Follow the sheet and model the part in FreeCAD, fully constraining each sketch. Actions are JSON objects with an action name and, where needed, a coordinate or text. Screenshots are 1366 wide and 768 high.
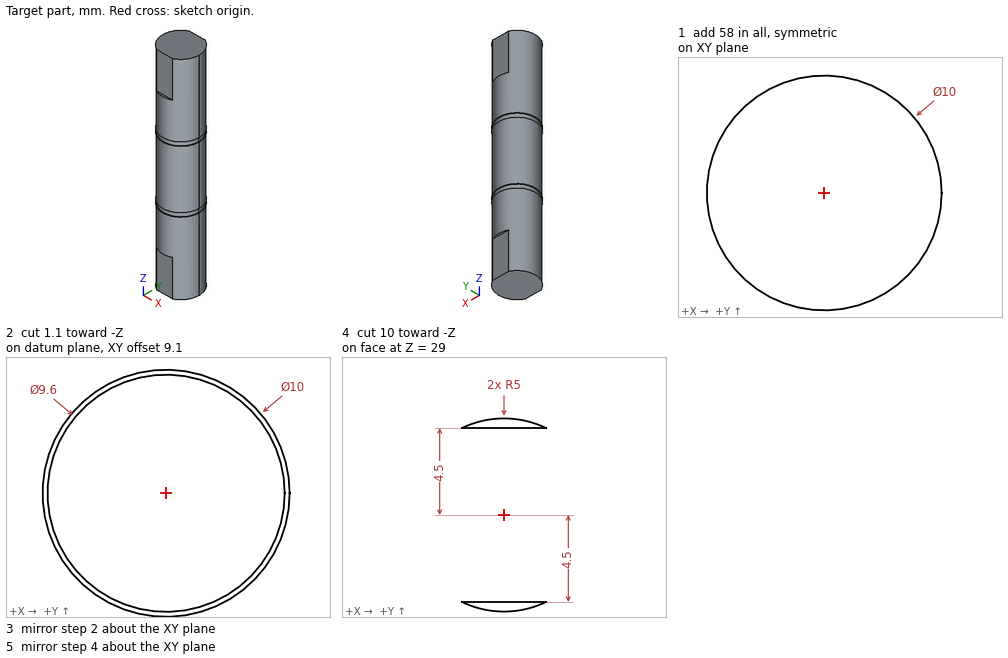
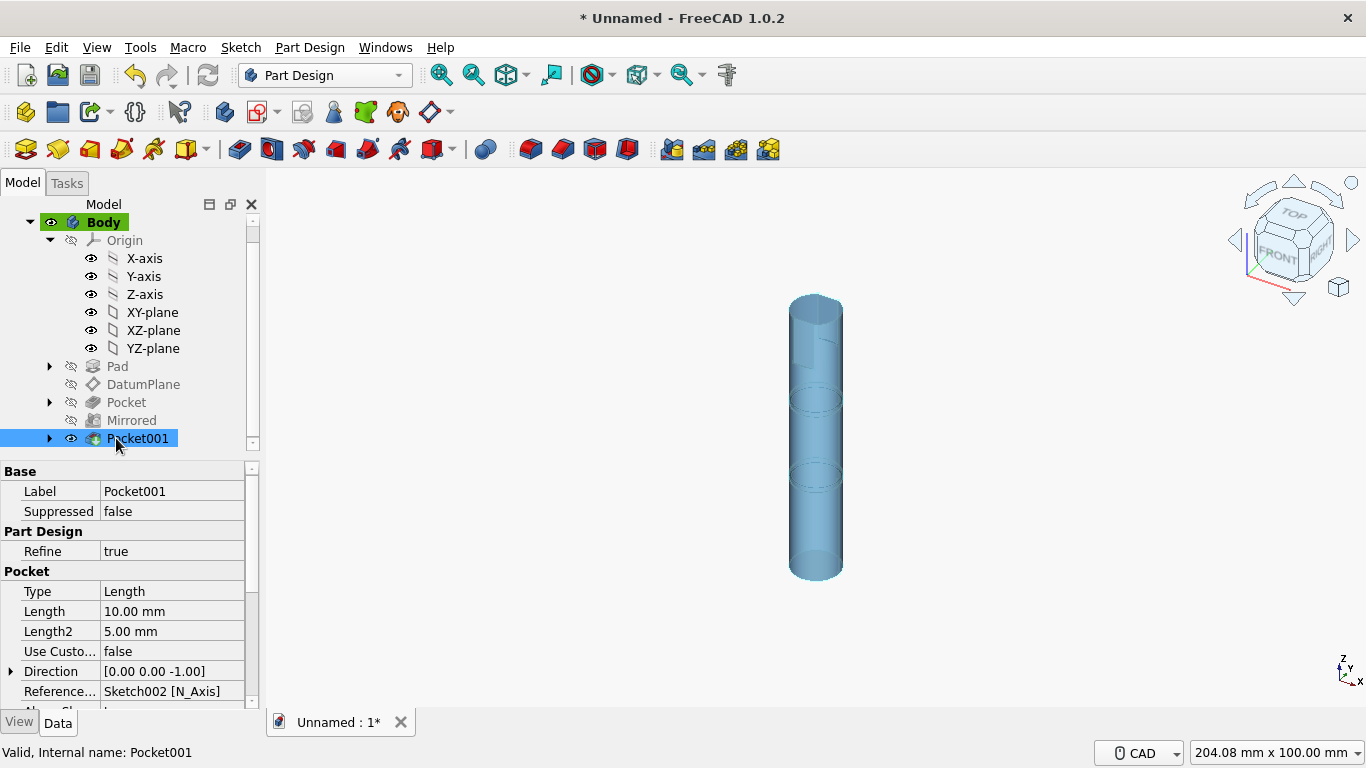
{"action": "left_click", "coordinate": [672, 150]}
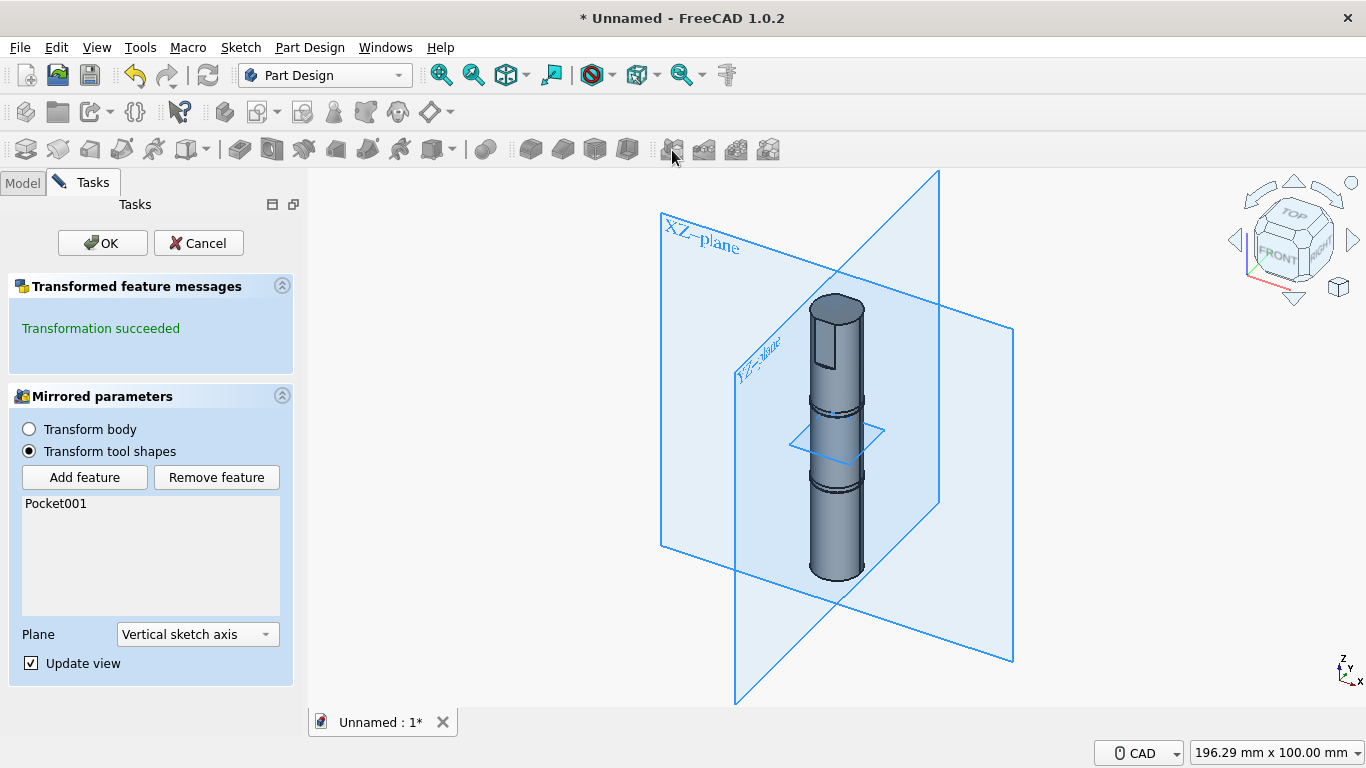
{"action": "left_click", "coordinate": [198, 634]}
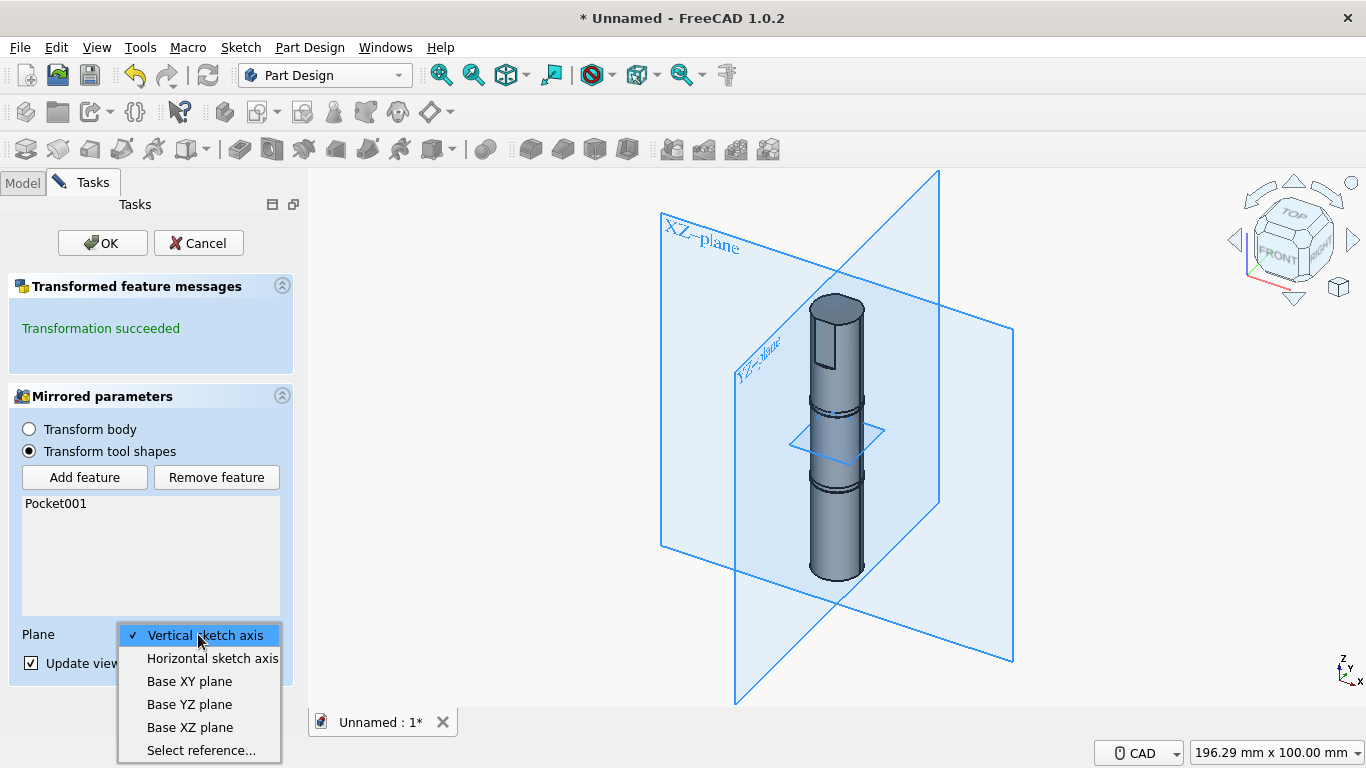
{"action": "left_click", "coordinate": [198, 682]}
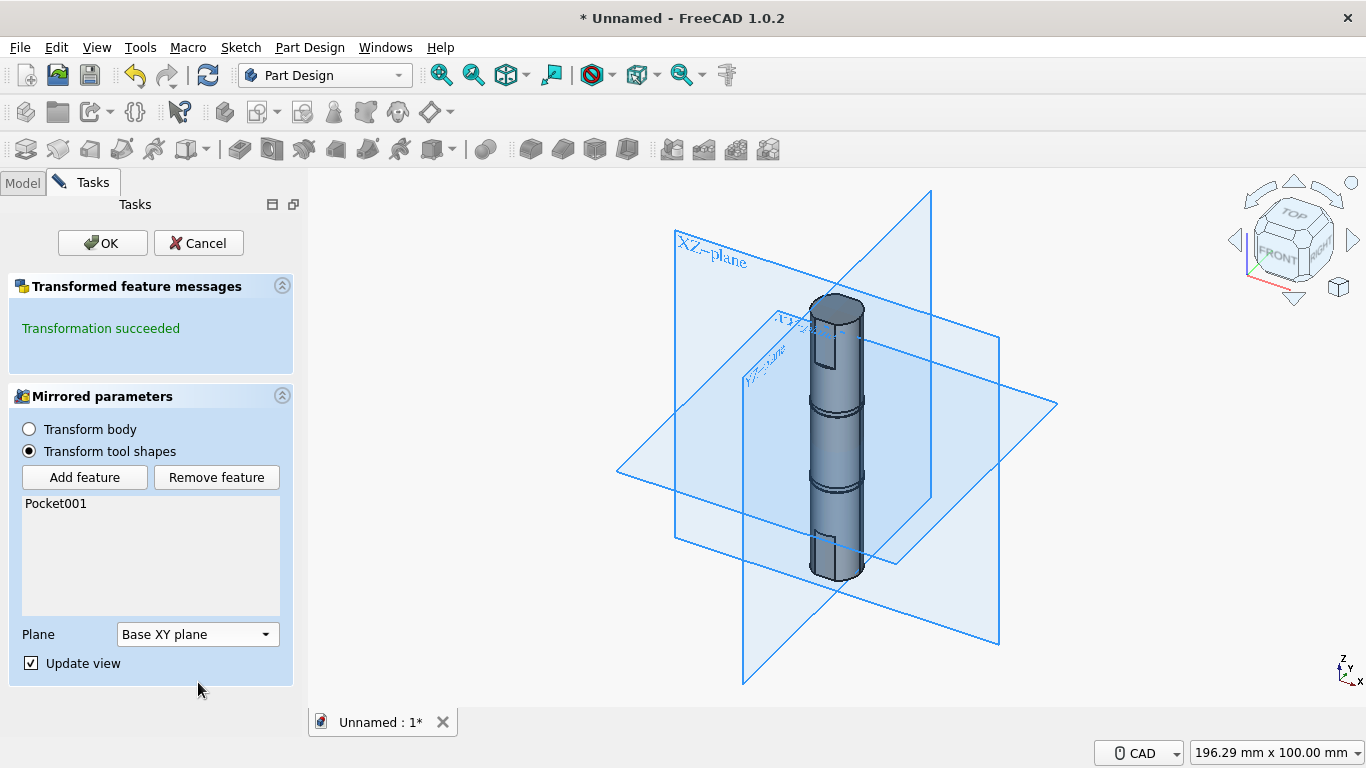
{"action": "left_click", "coordinate": [103, 243]}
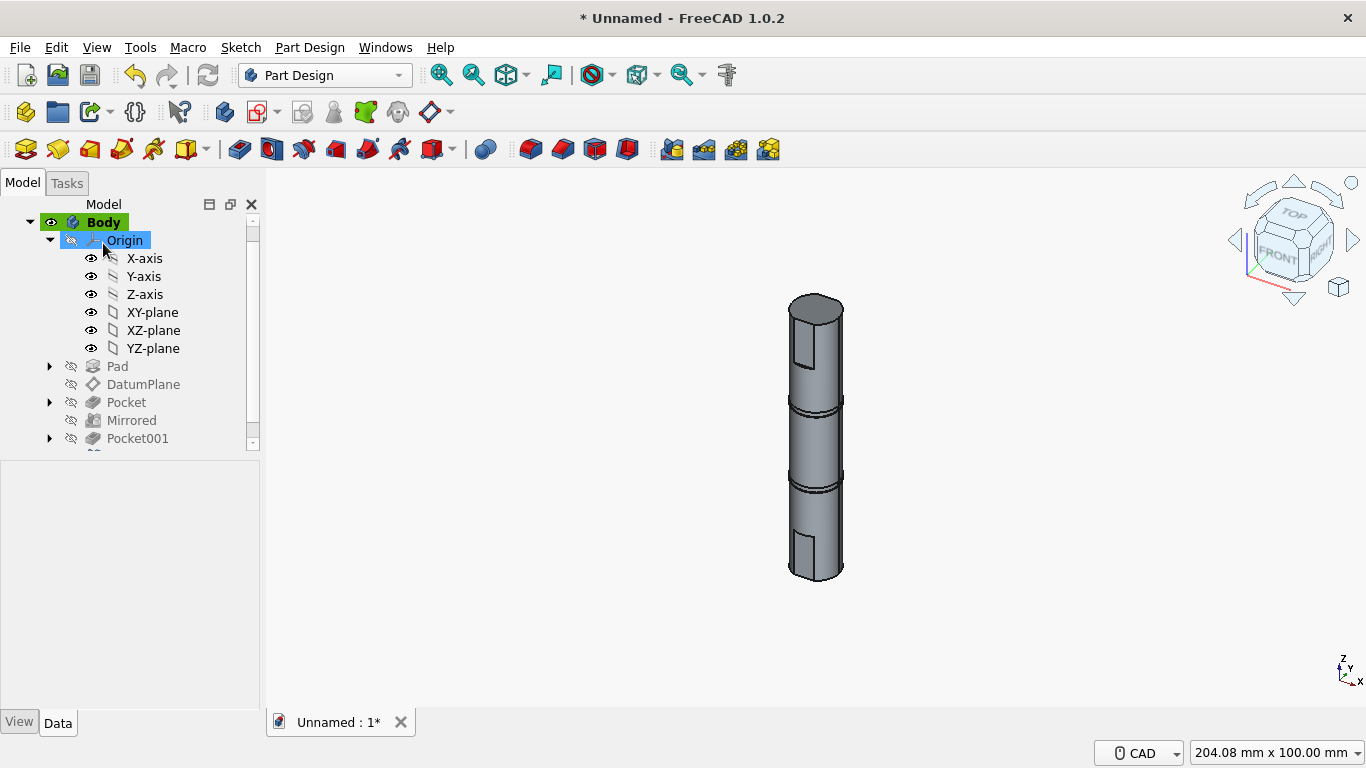
{"action": "key", "text": "0"}